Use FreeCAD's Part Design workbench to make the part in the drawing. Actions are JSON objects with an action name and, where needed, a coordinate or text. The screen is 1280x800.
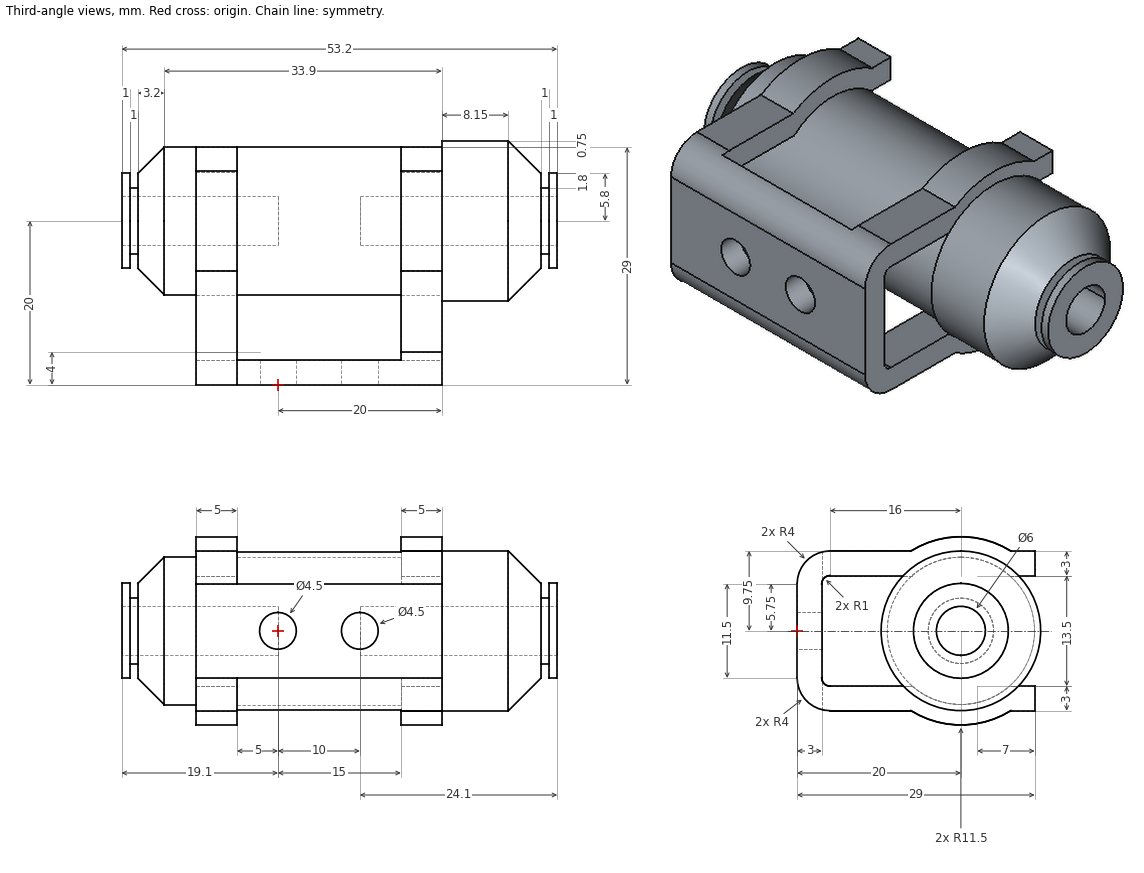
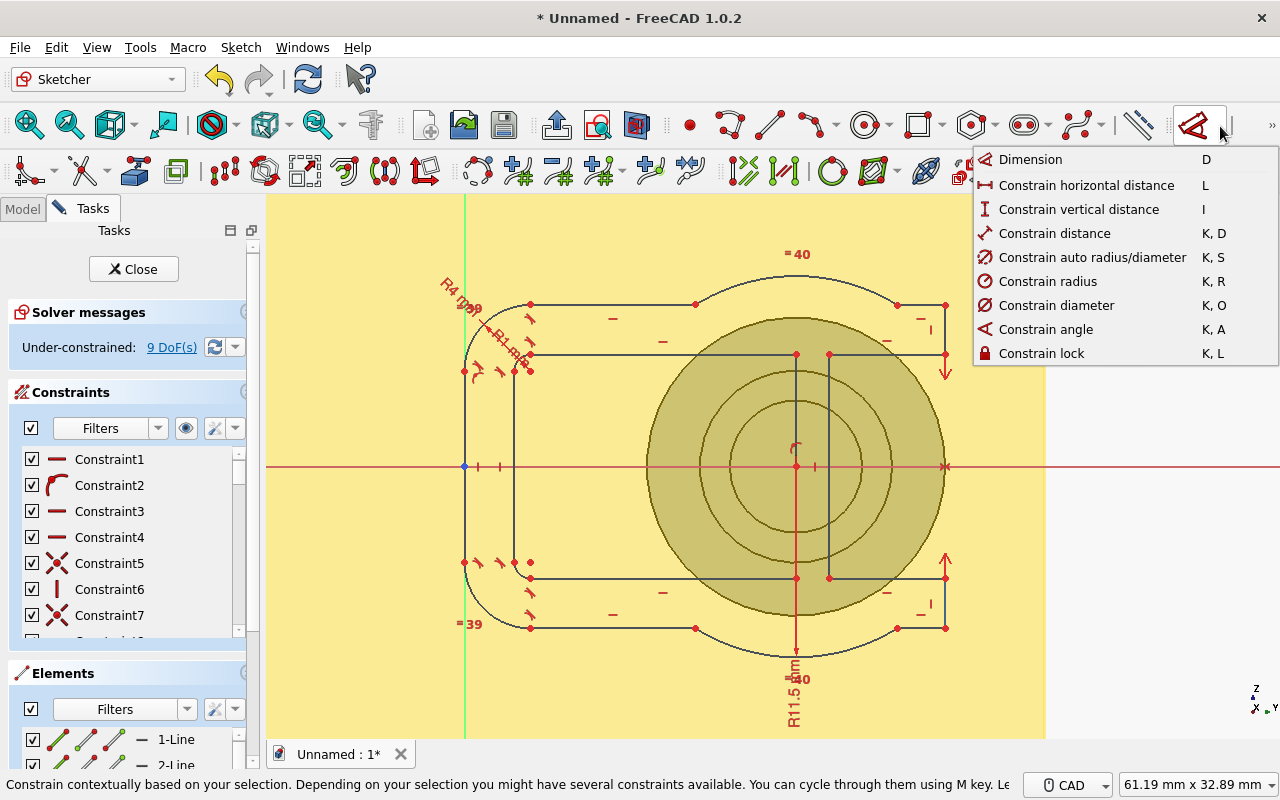
{"action": "left_click", "coordinate": [1126, 209]}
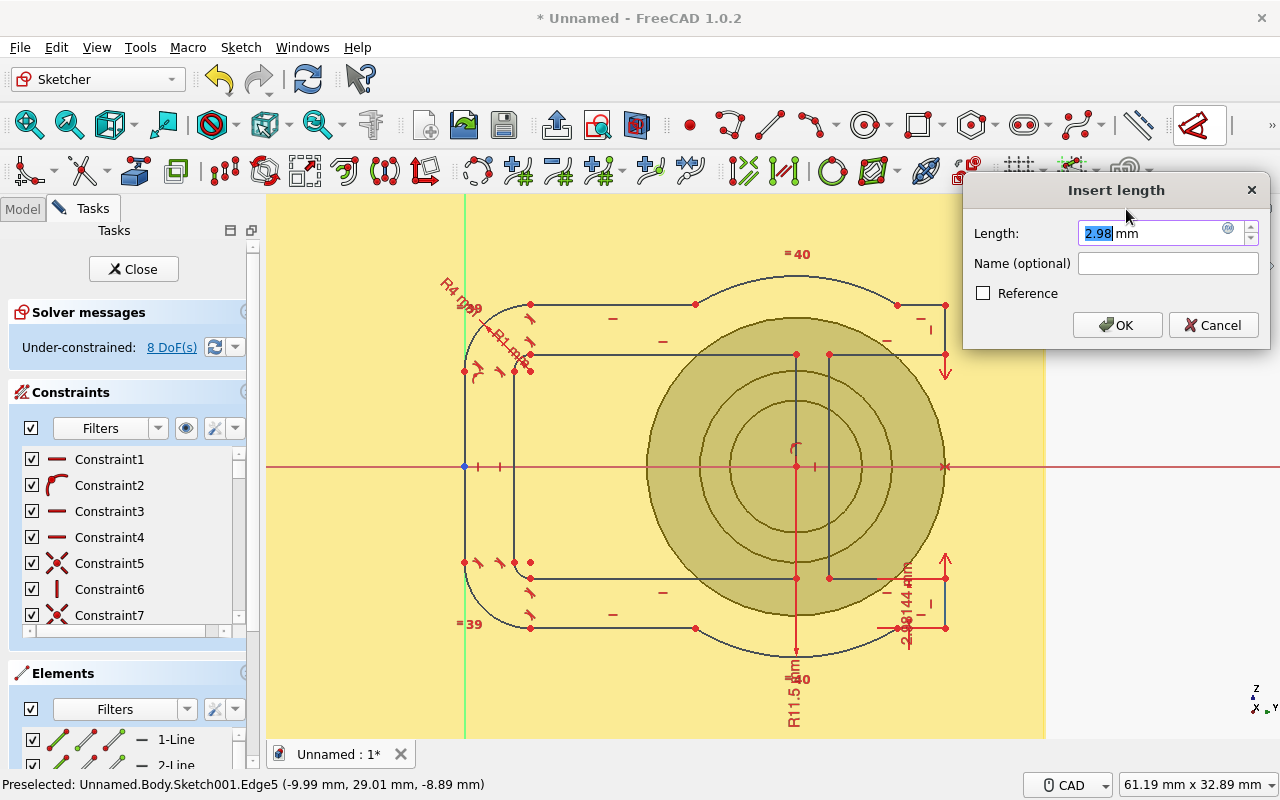
{"action": "type", "text": "3"}
{"action": "key", "text": "Return"}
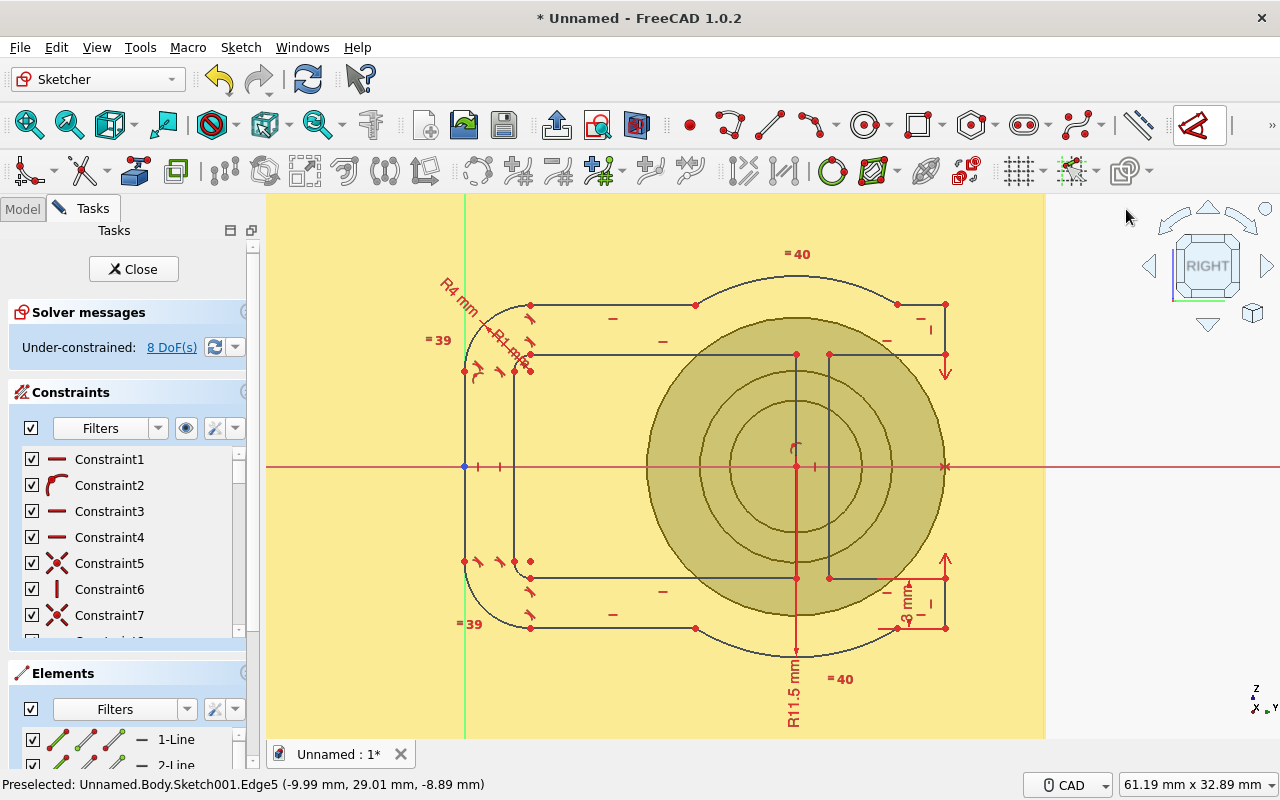
{"action": "left_click", "coordinate": [911, 579]}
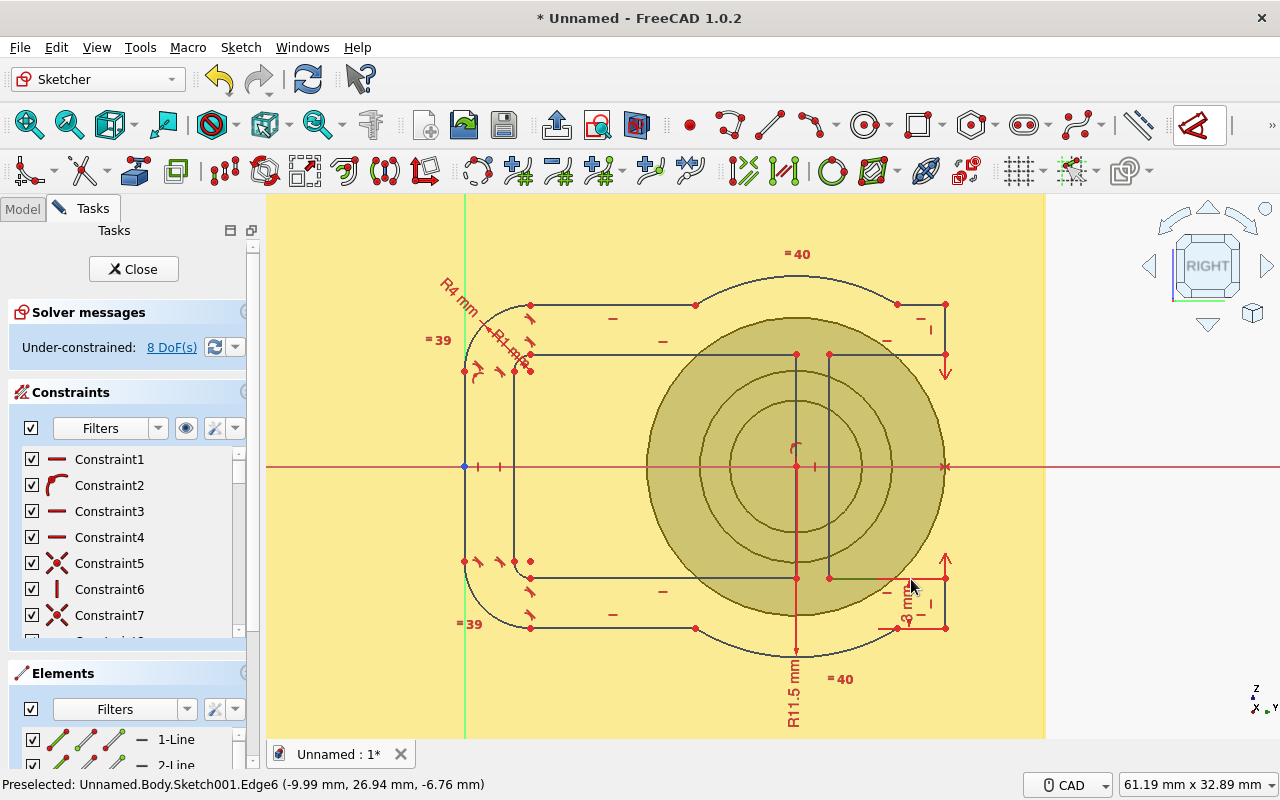
{"action": "left_click", "coordinate": [1220, 126]}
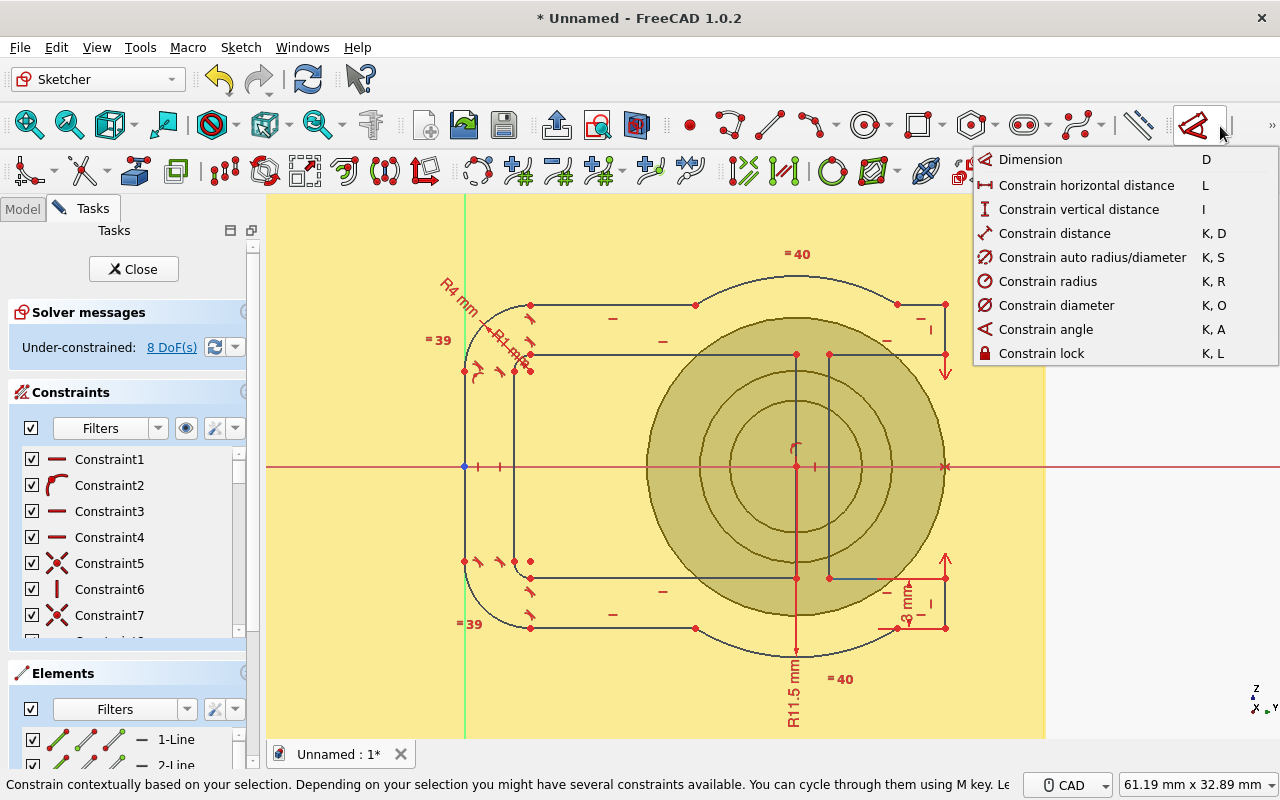
{"action": "left_click", "coordinate": [1126, 185]}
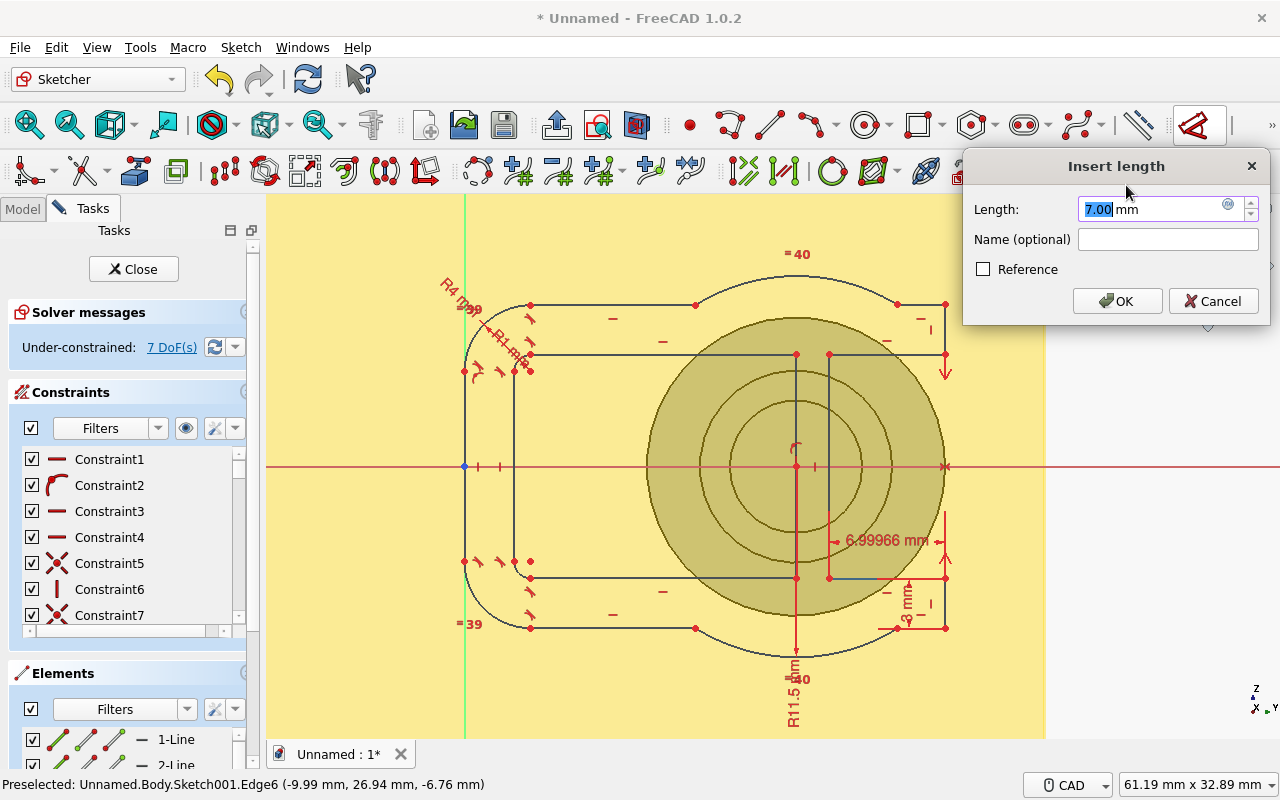
{"action": "type", "text": "7"}
{"action": "key", "text": "Return"}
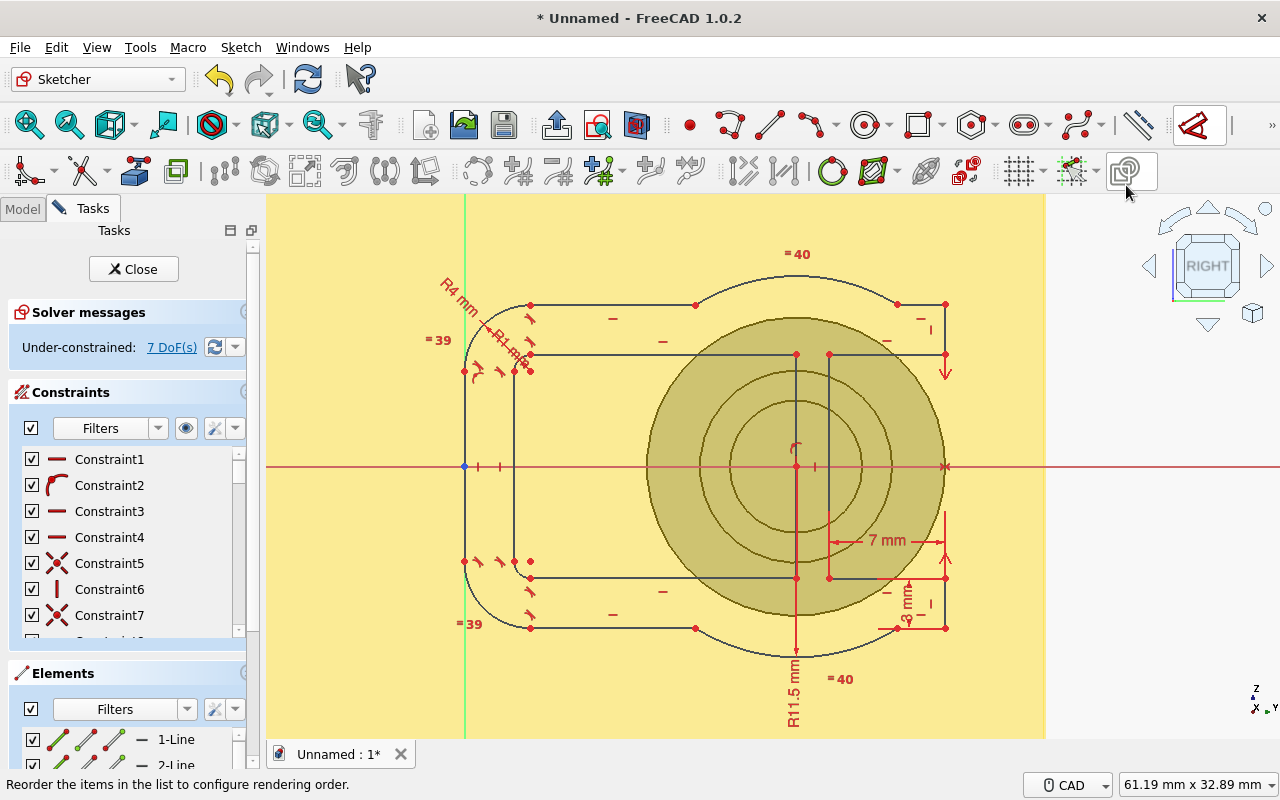
{"action": "left_click", "coordinate": [945, 340]}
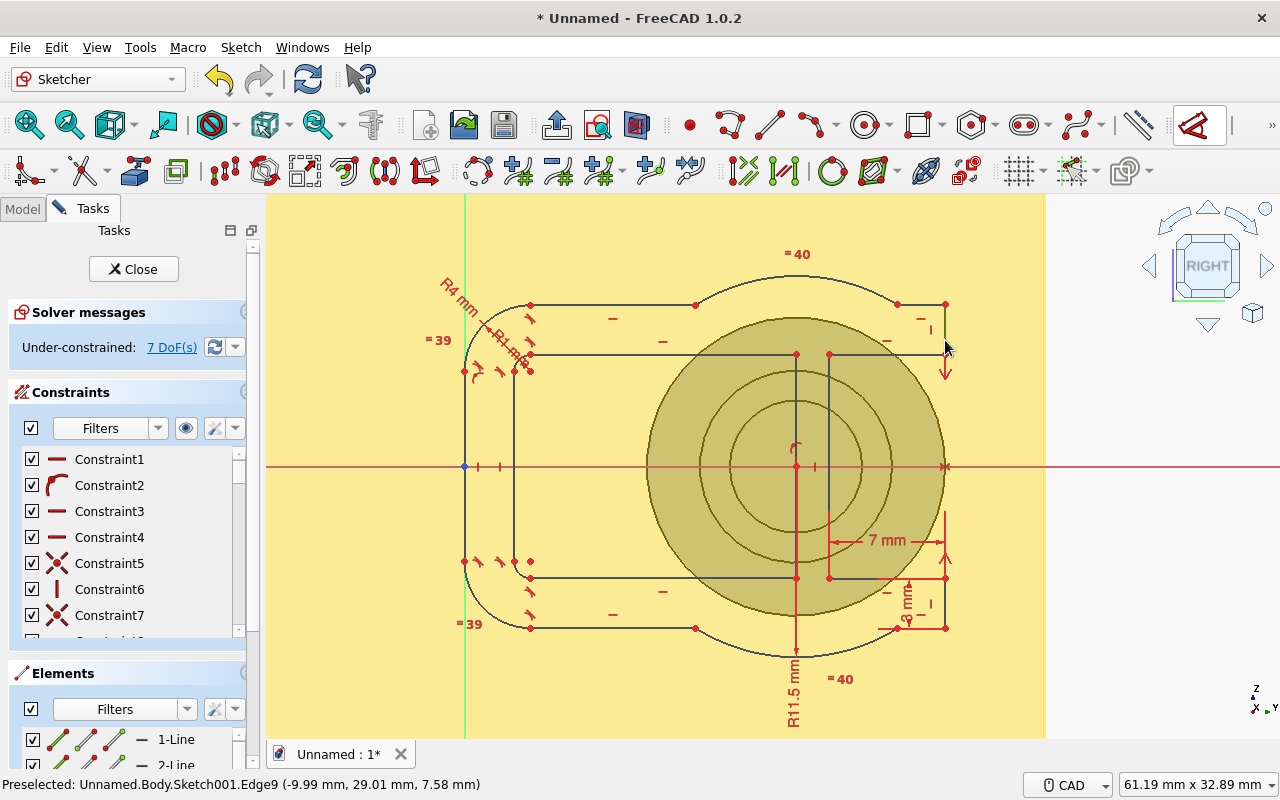
{"action": "key", "text": "i"}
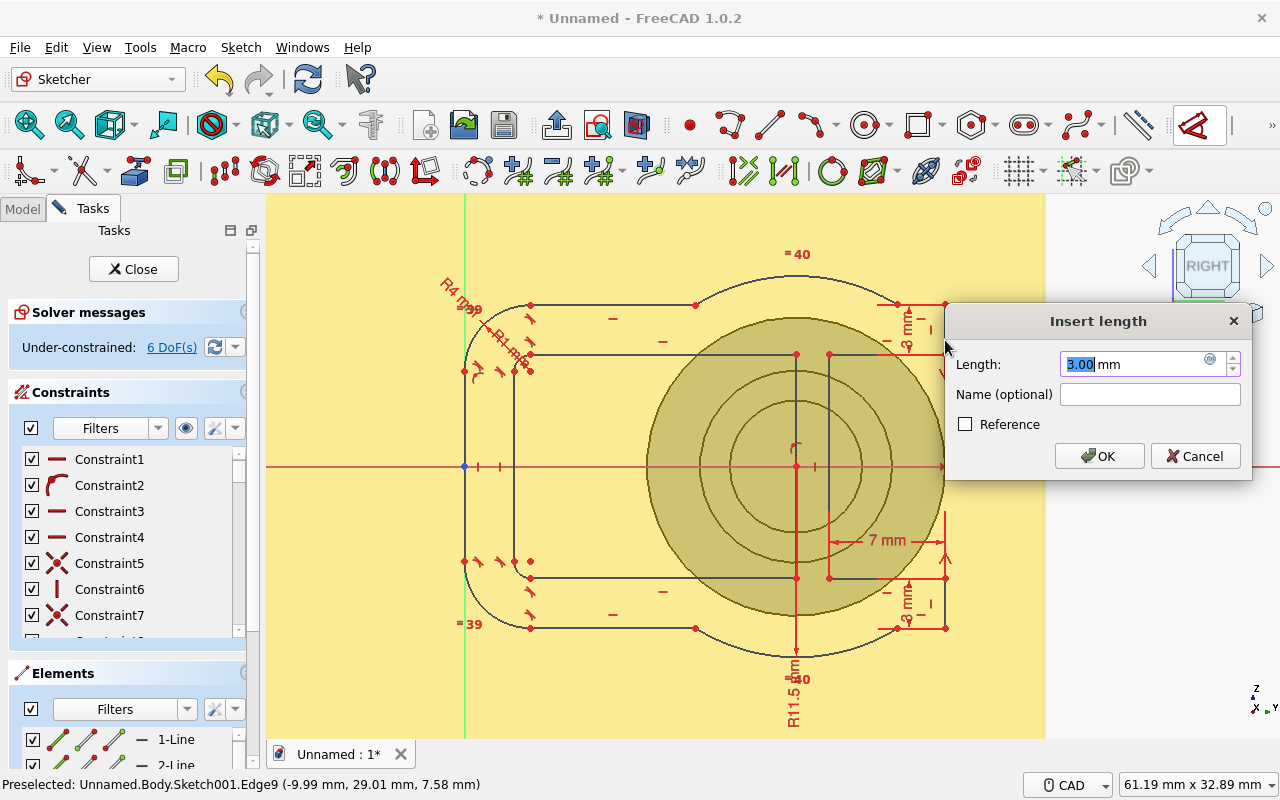
{"action": "type", "text": "3"}
{"action": "key", "text": "Return"}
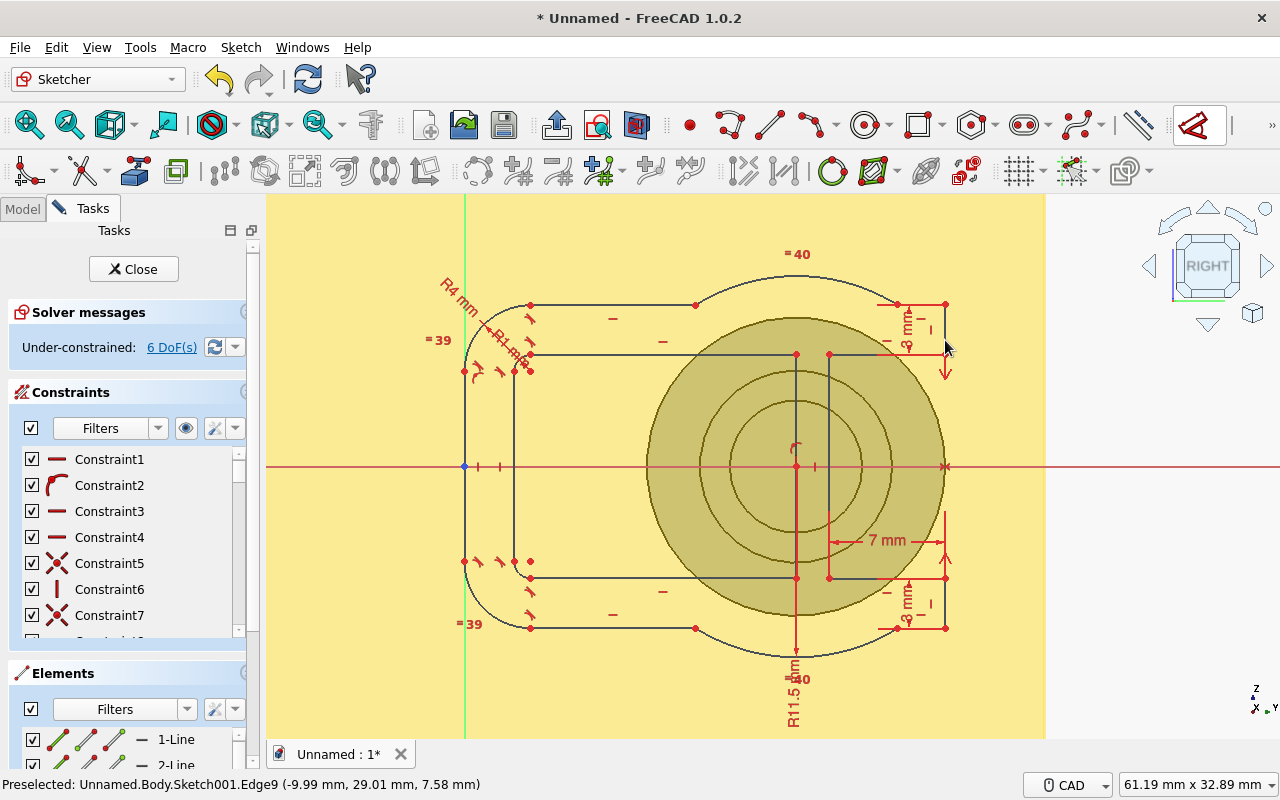
{"action": "left_click", "coordinate": [611, 355]}